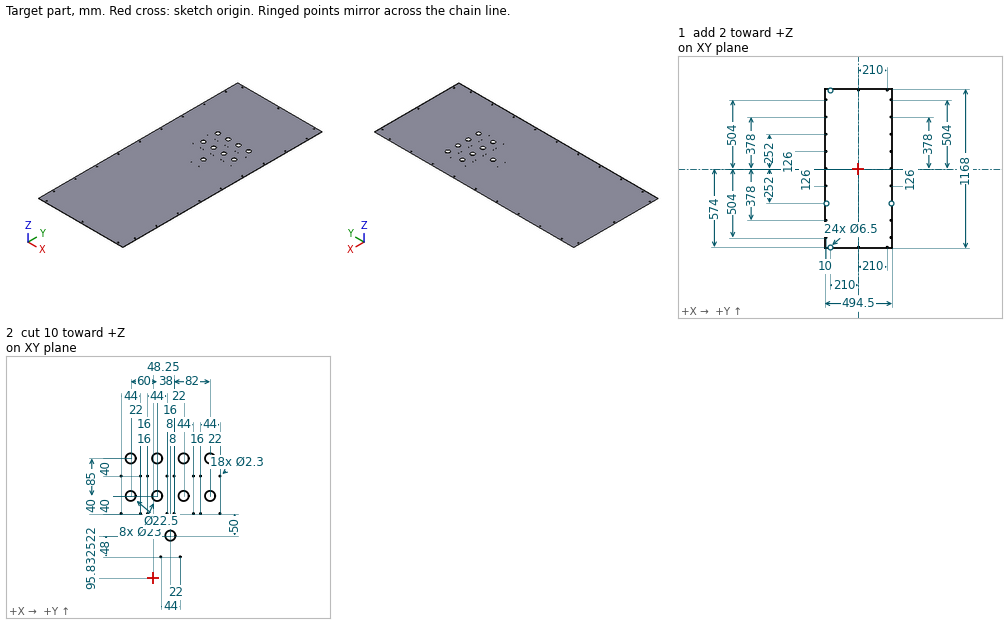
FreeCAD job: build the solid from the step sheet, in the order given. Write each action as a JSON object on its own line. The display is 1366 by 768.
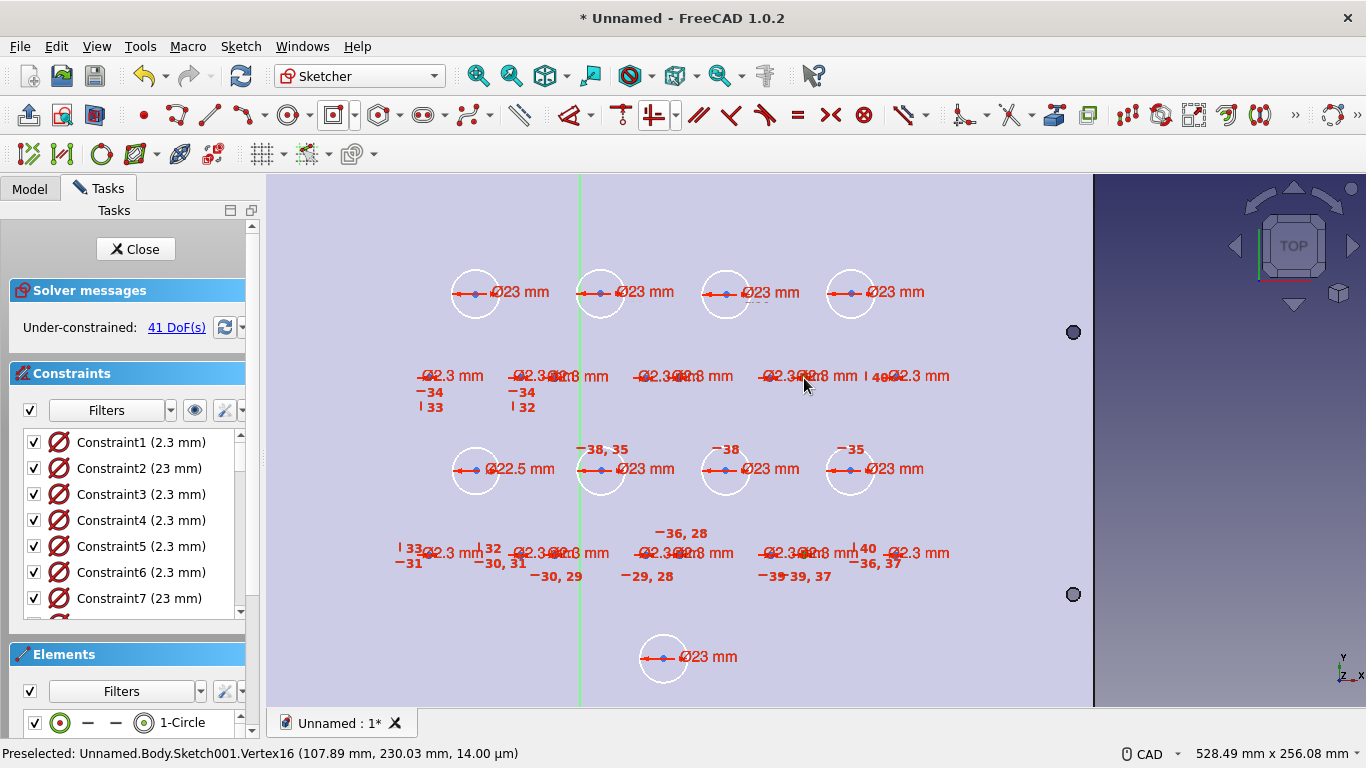
{"action": "key", "text": "v"}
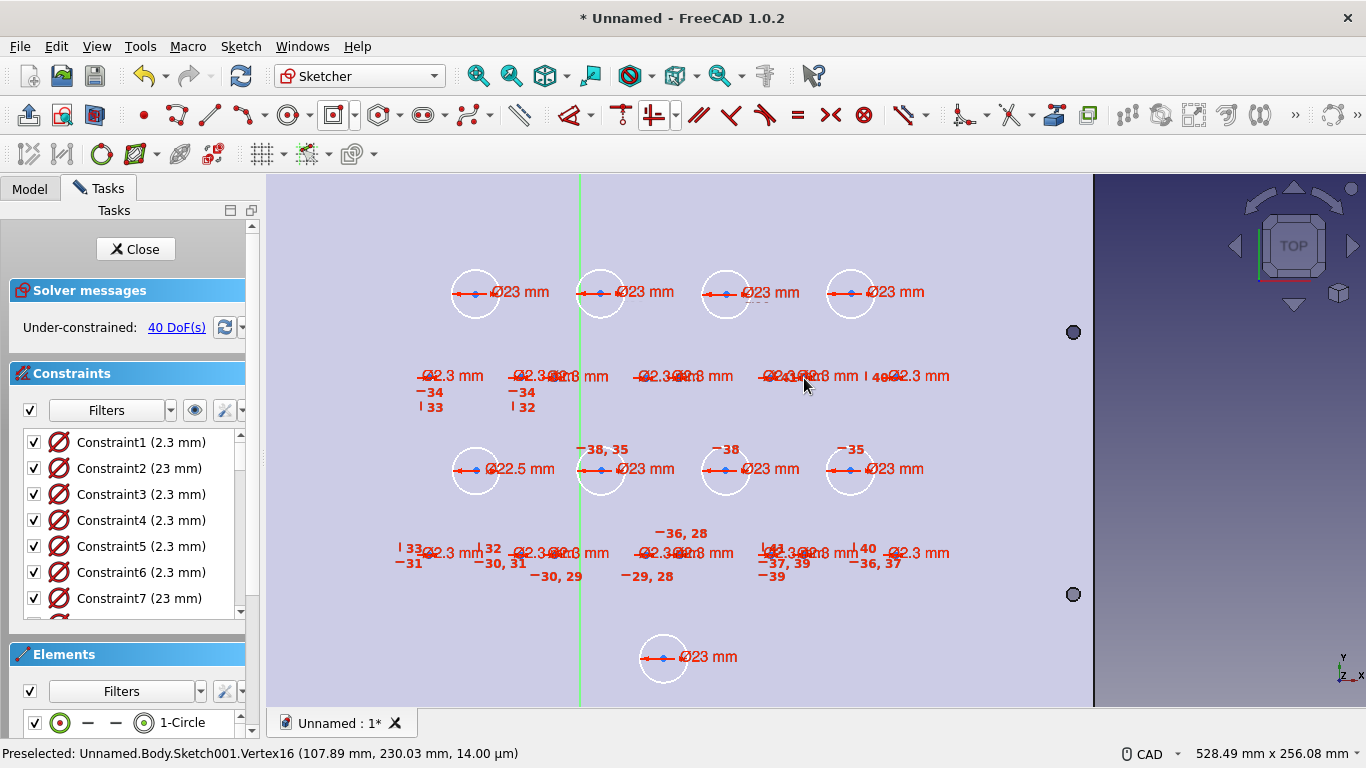
{"action": "left_click", "coordinate": [896, 378]}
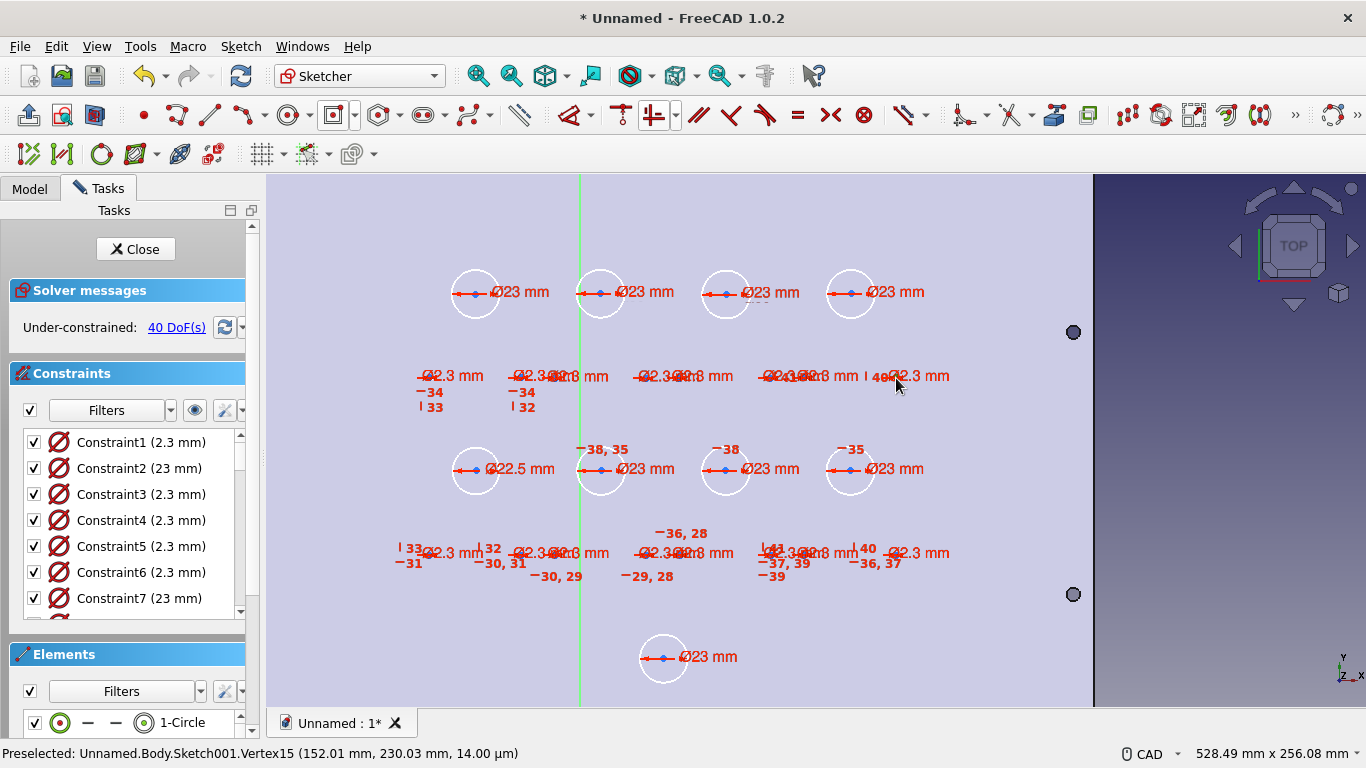
{"action": "left_click", "coordinate": [805, 378]}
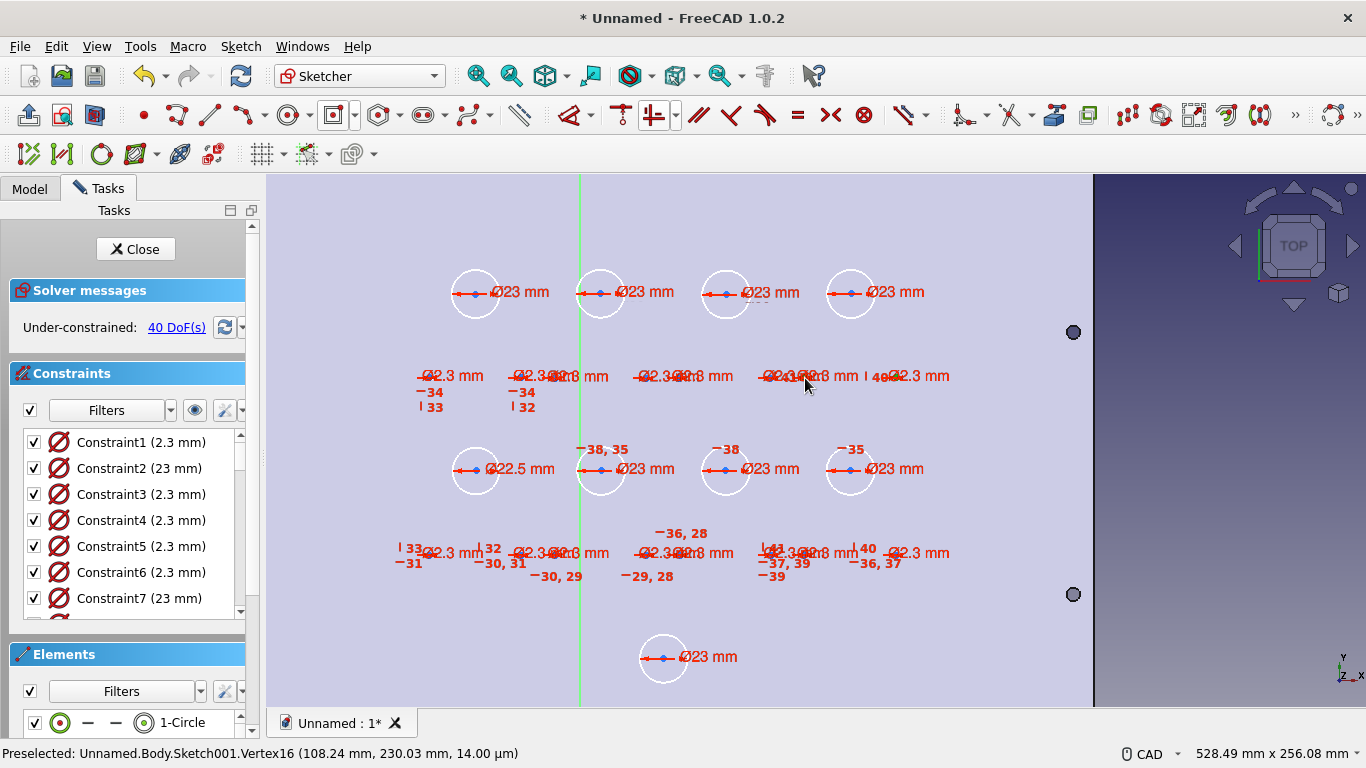
{"action": "key", "text": "h"}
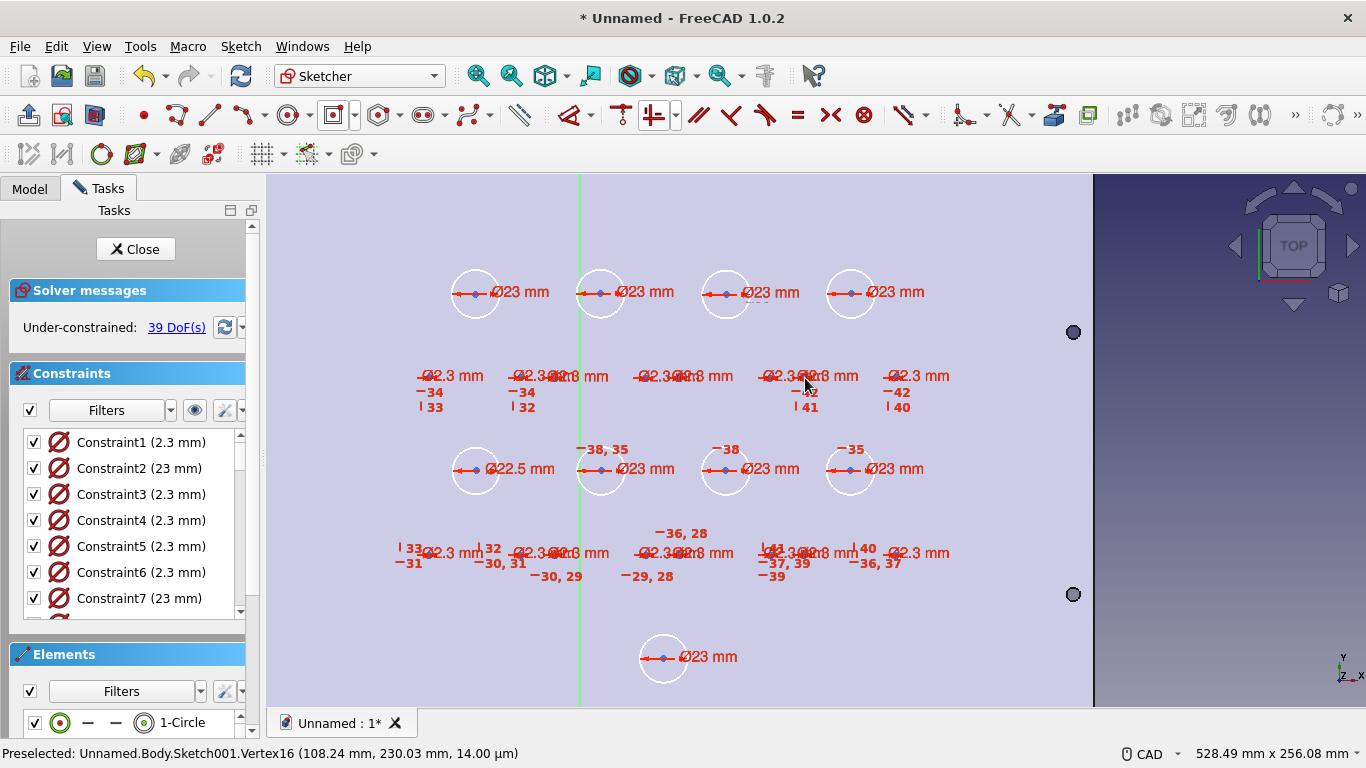
{"action": "left_click", "coordinate": [726, 471]}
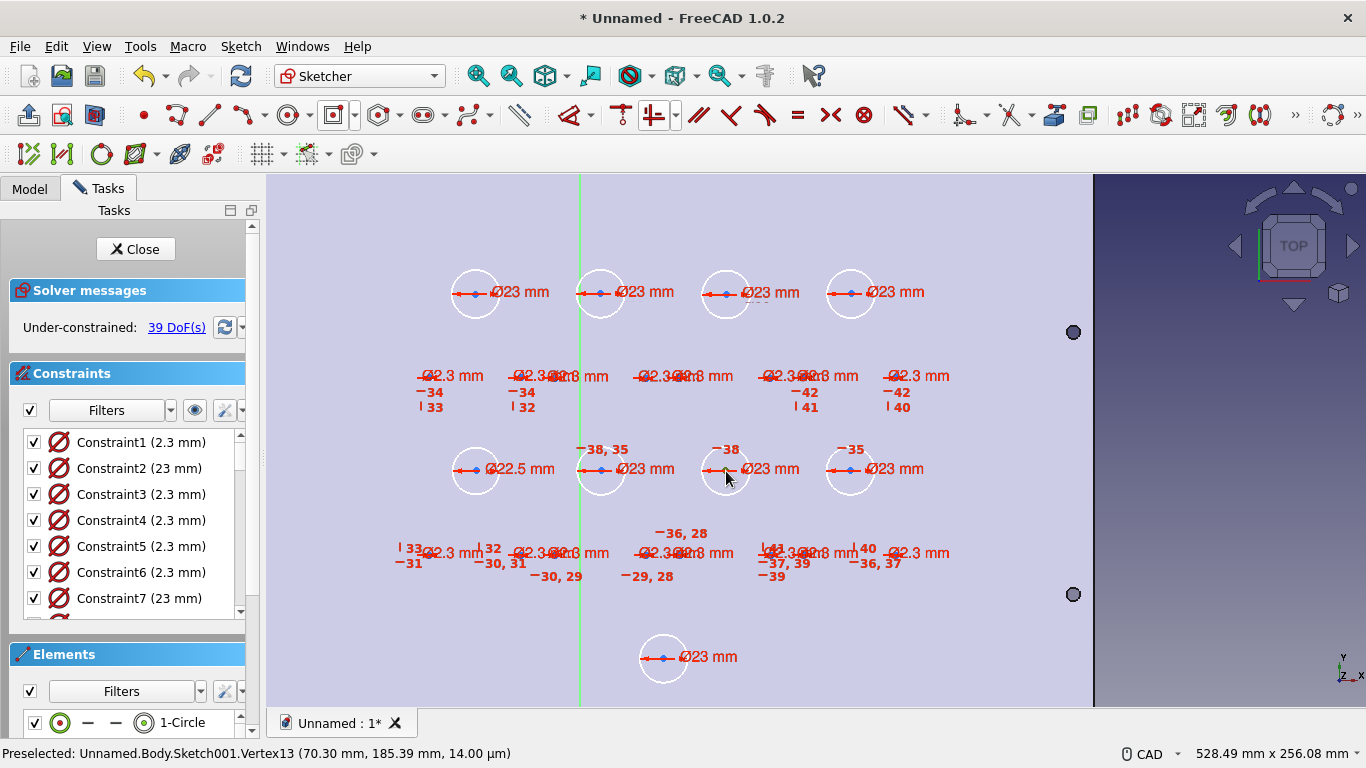
{"action": "left_click", "coordinate": [726, 295]}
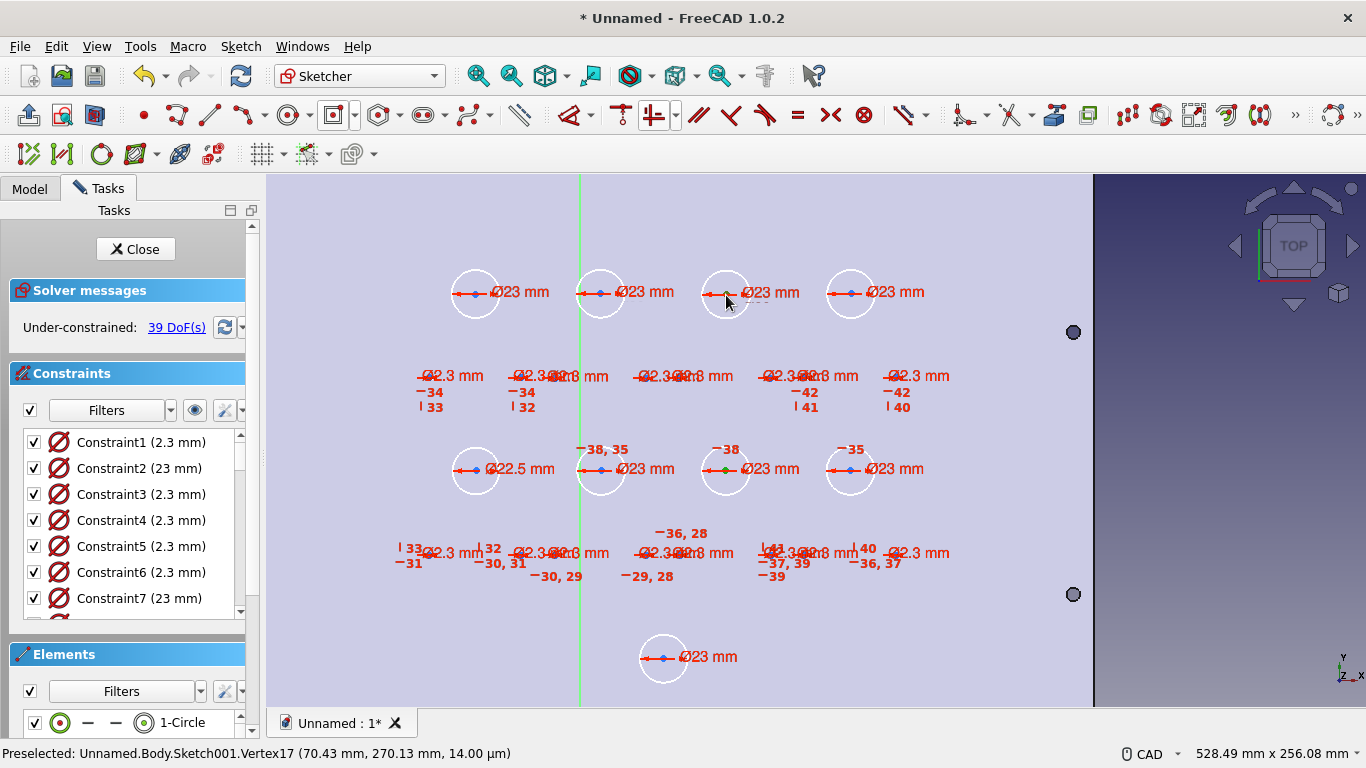
{"action": "key", "text": "v"}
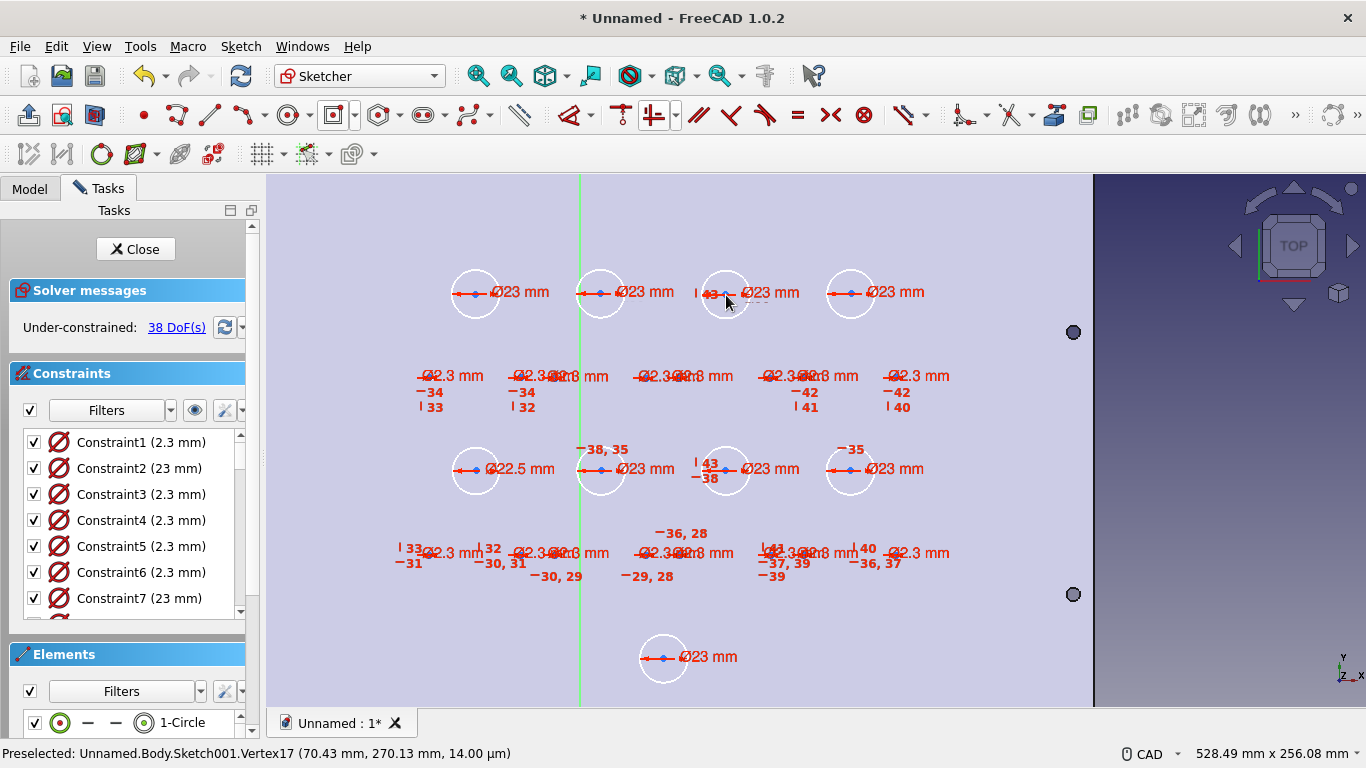
{"action": "left_click", "coordinate": [771, 555]}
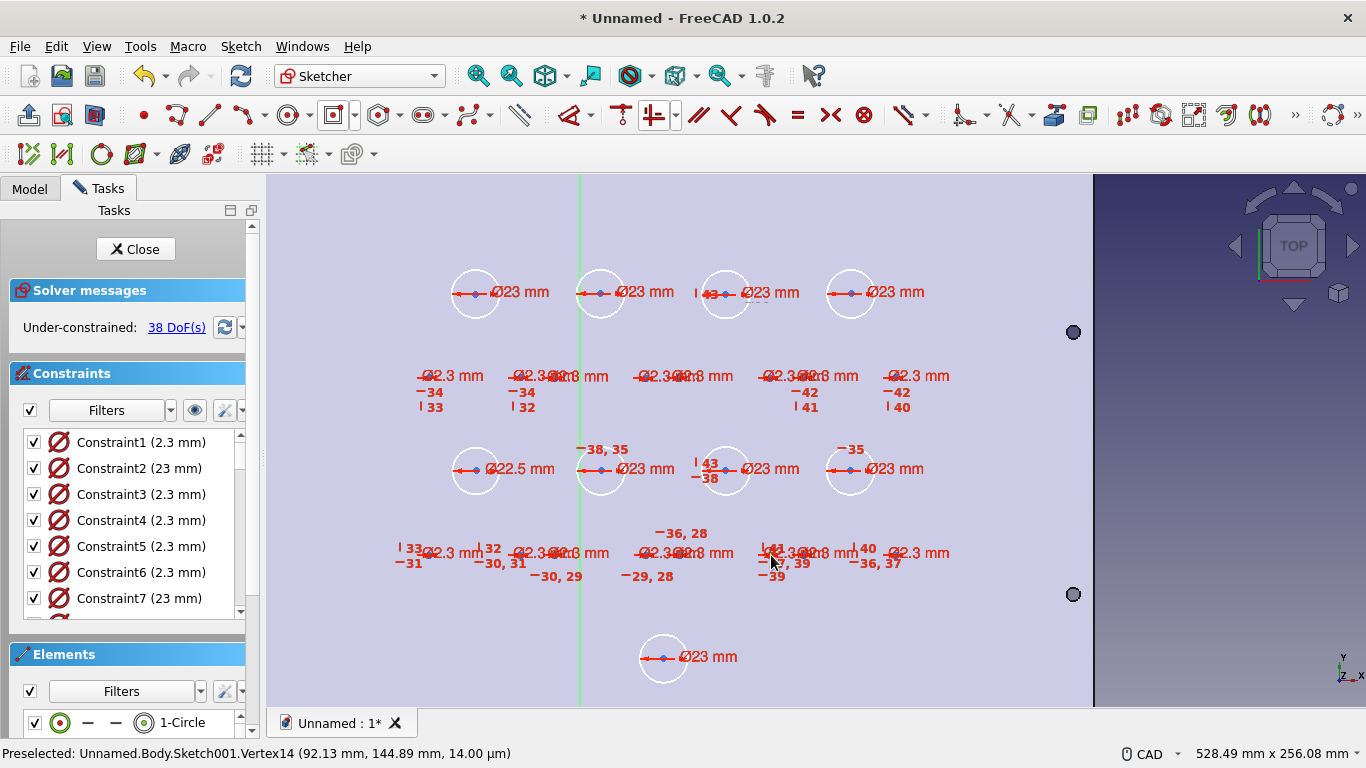
{"action": "left_click", "coordinate": [771, 378]}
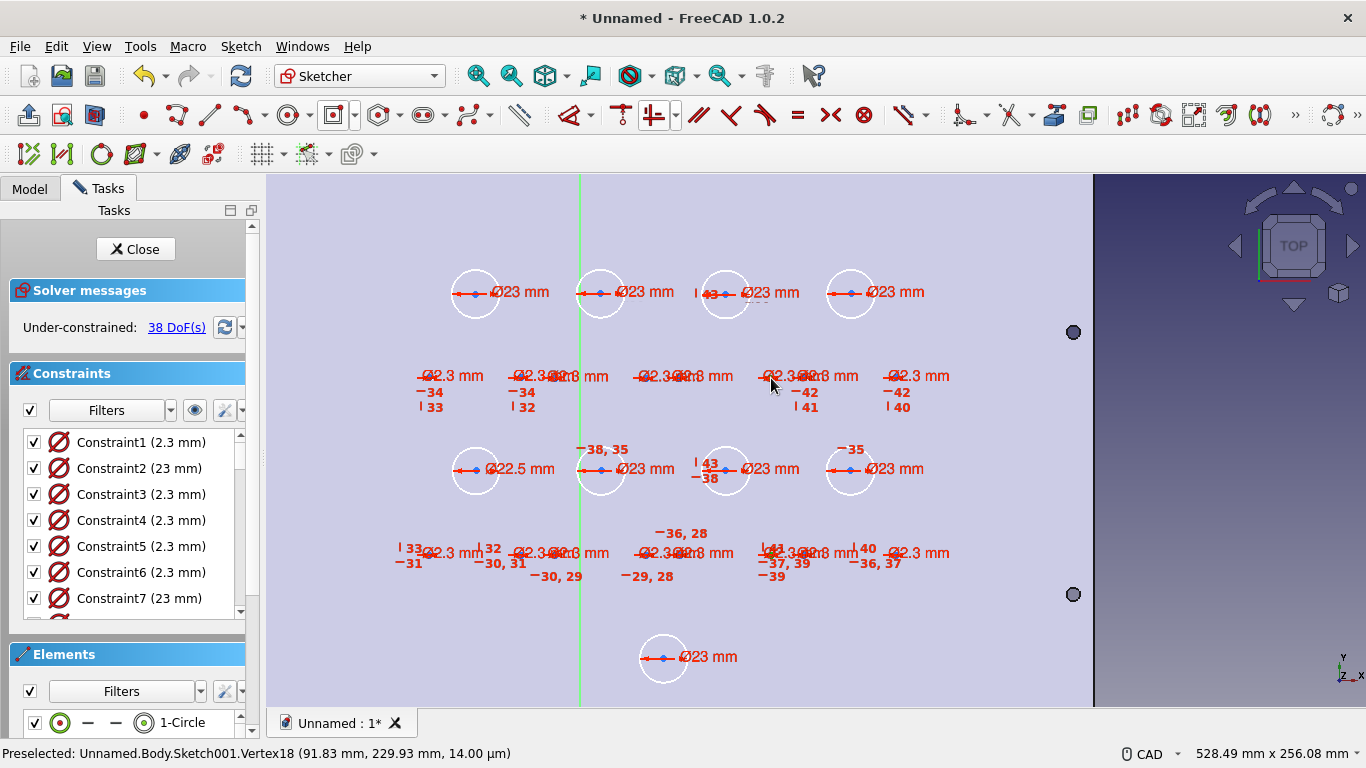
{"action": "left_click", "coordinate": [676, 116]}